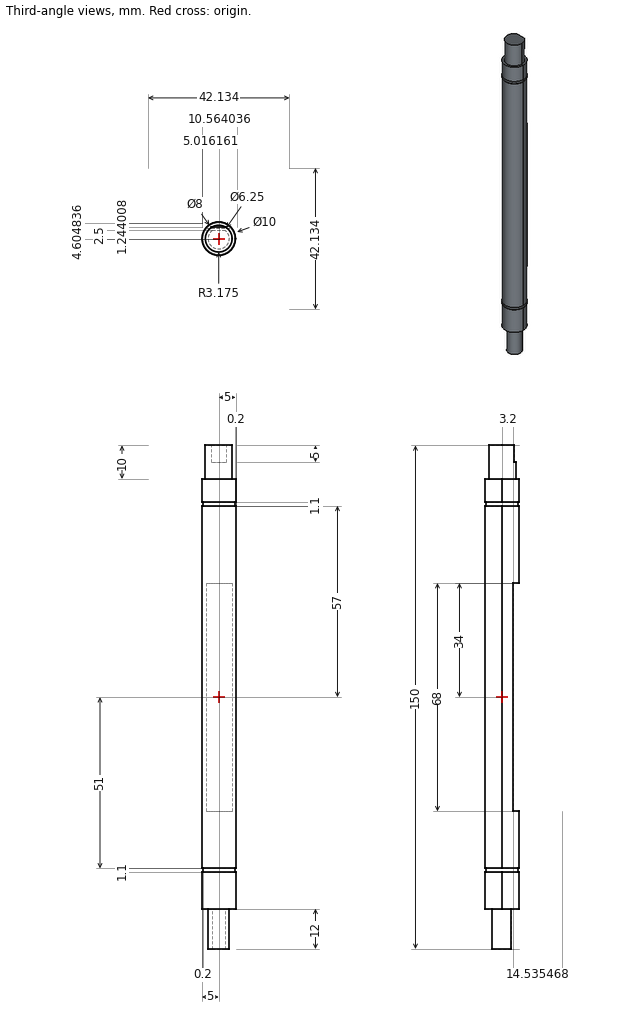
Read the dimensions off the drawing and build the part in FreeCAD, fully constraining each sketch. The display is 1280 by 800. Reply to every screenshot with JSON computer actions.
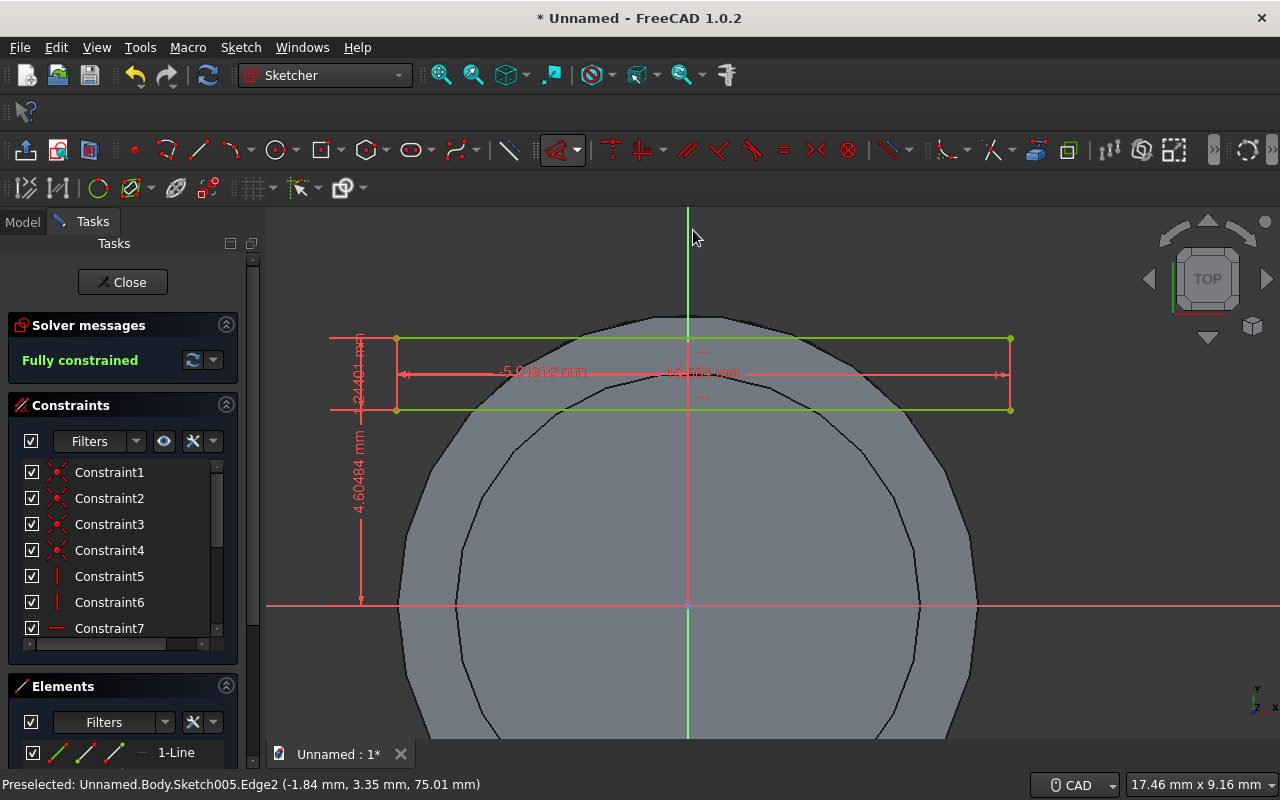
{"action": "left_click", "coordinate": [123, 282]}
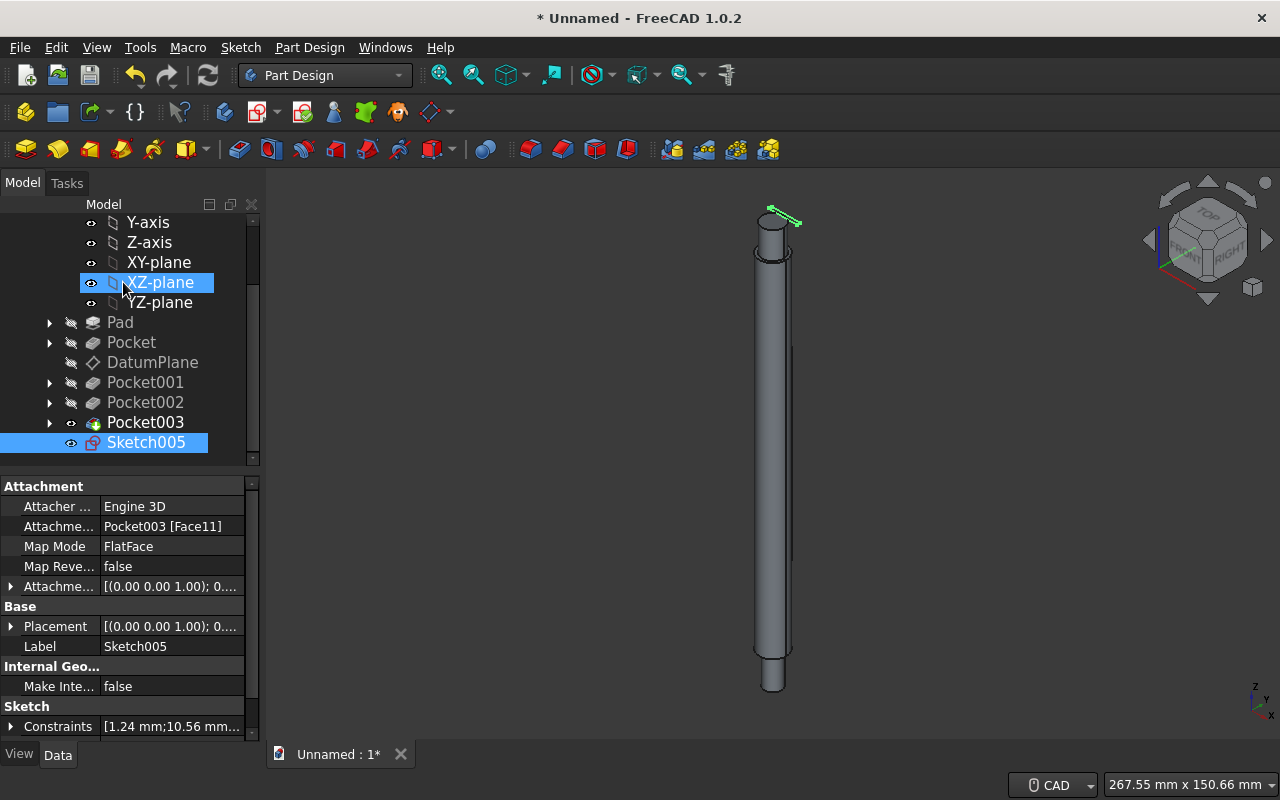
{"action": "left_click", "coordinate": [240, 150]}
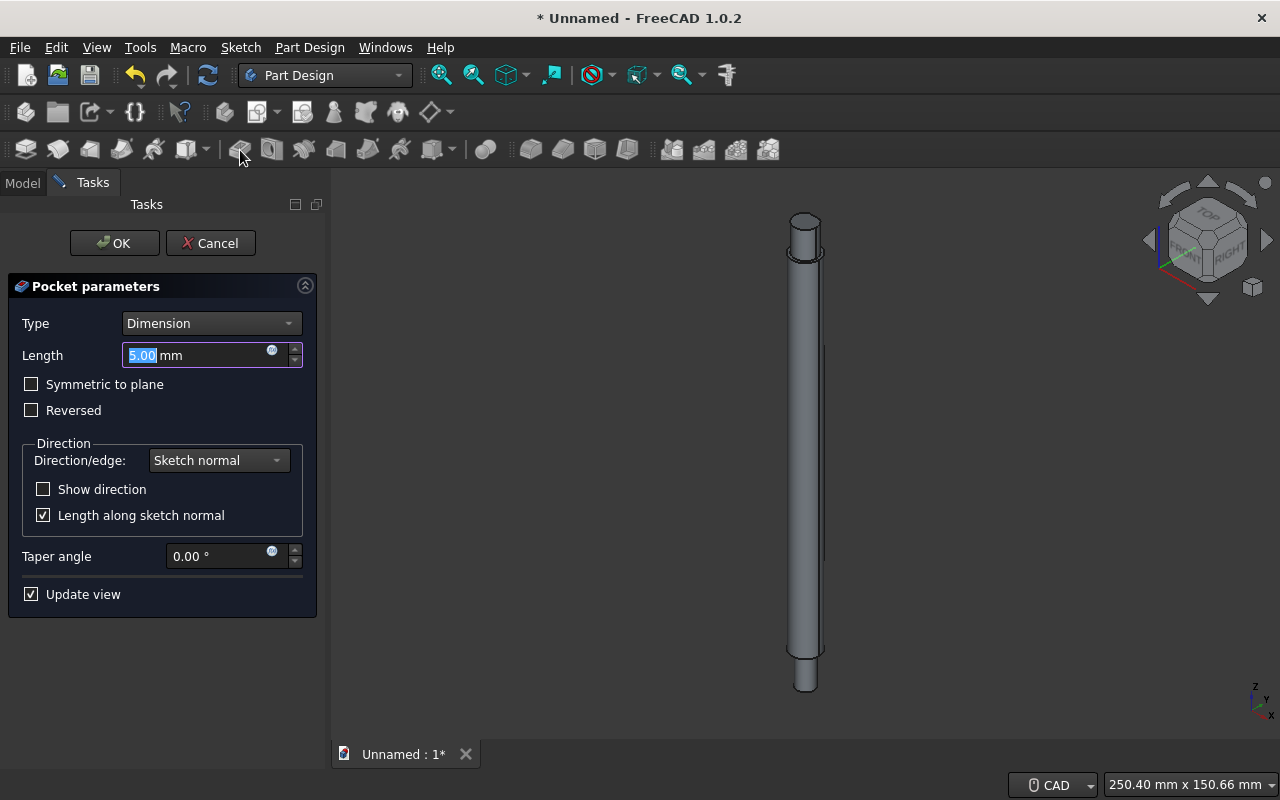
{"action": "type", "text": "5"}
{"action": "key", "text": "Tab"}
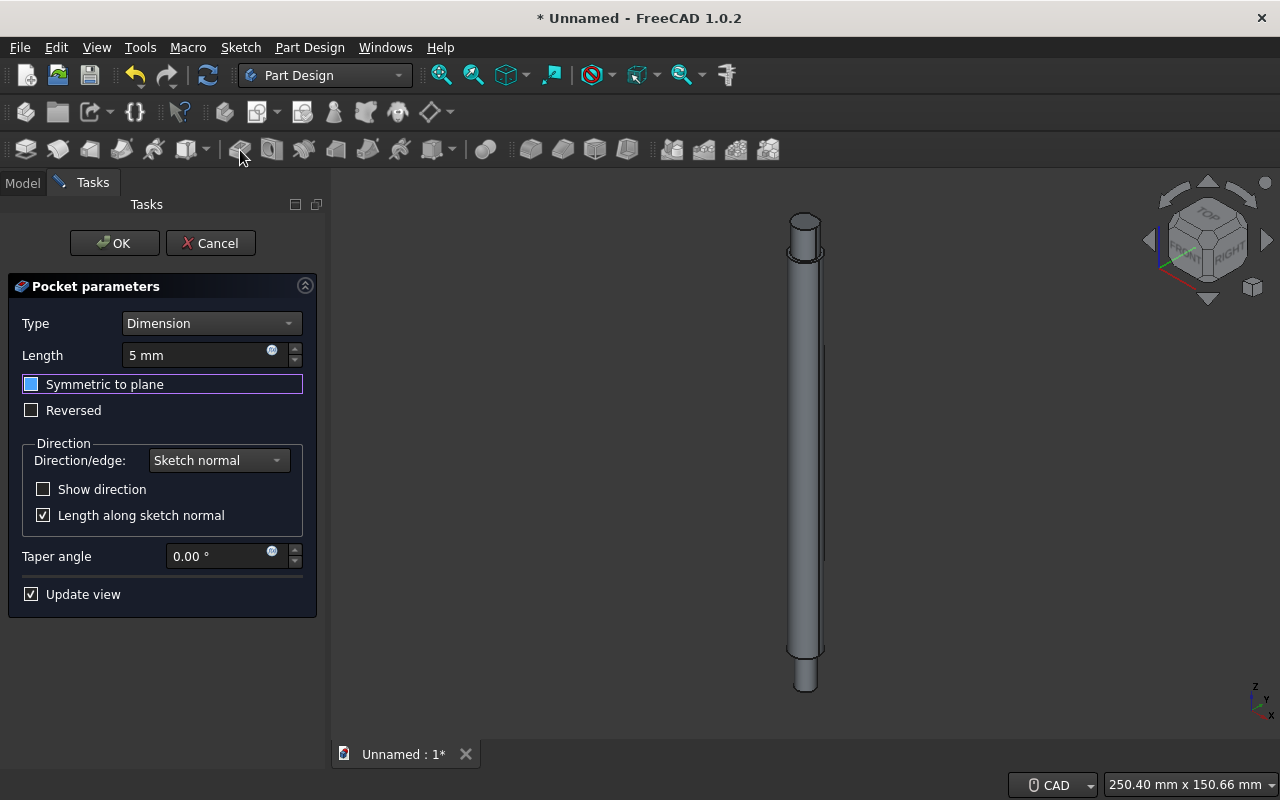
{"action": "left_click", "coordinate": [115, 243]}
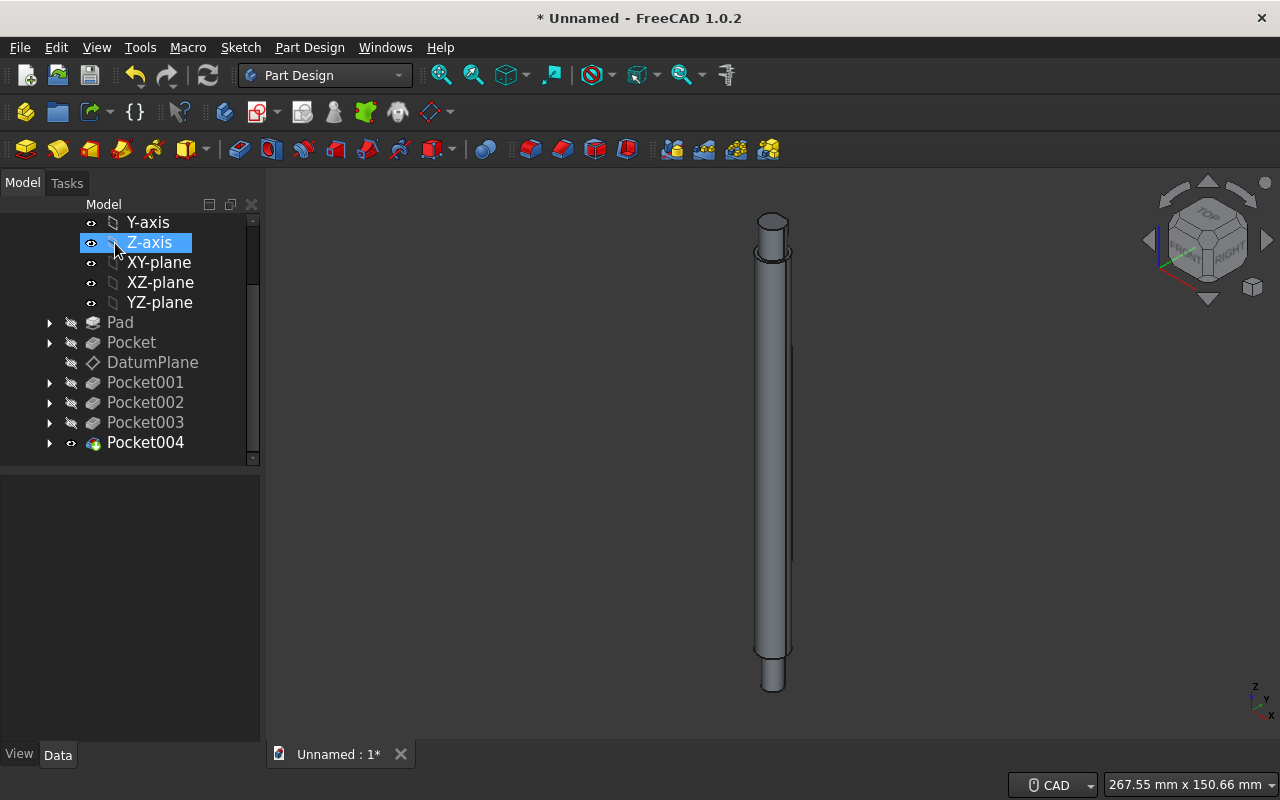
{"action": "left_click", "coordinate": [258, 112]}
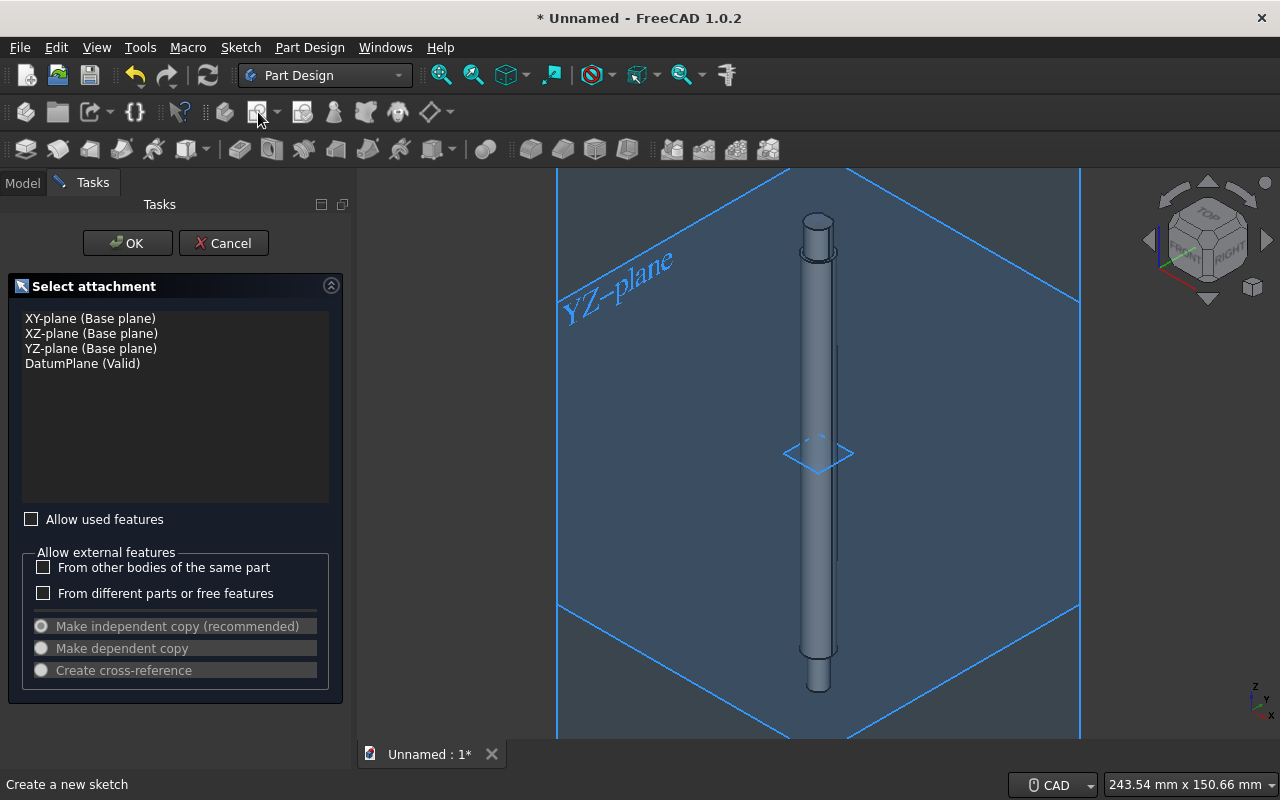
{"action": "left_click", "coordinate": [82, 334]}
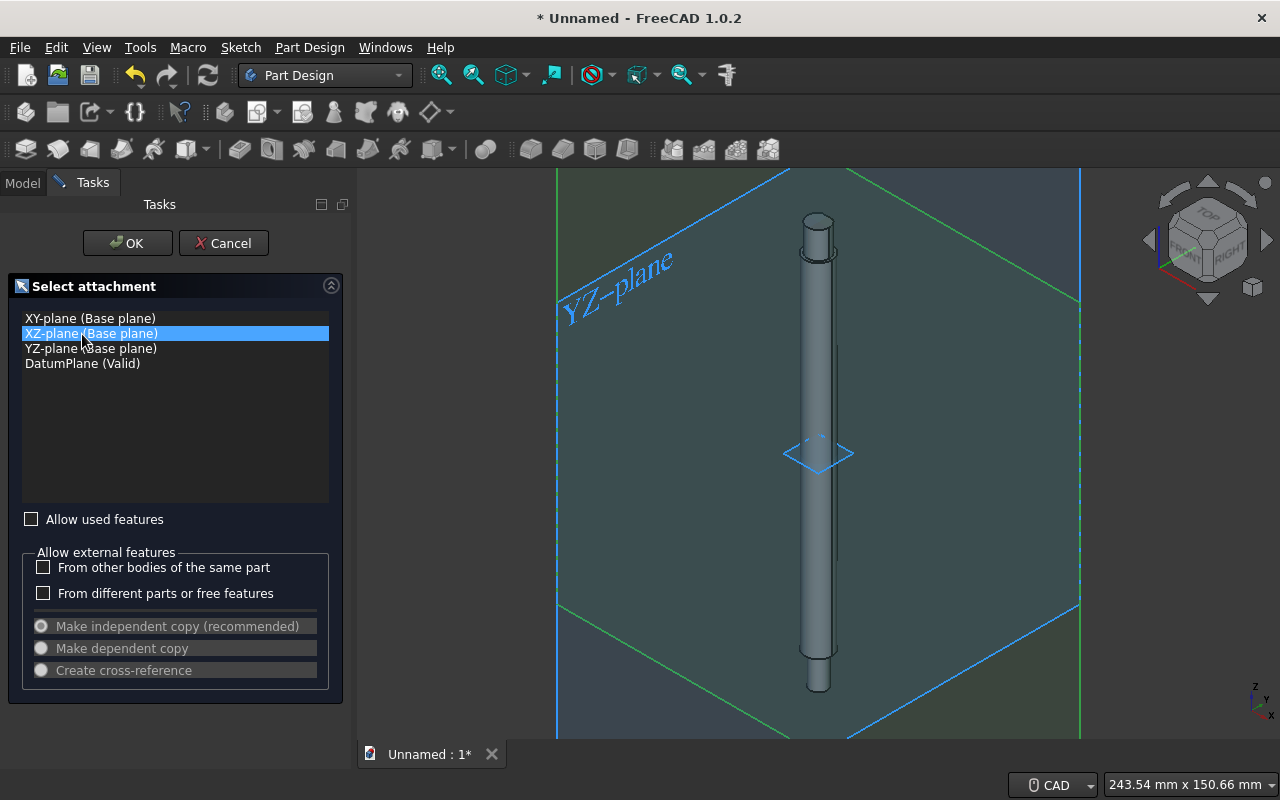
{"action": "left_click", "coordinate": [128, 243]}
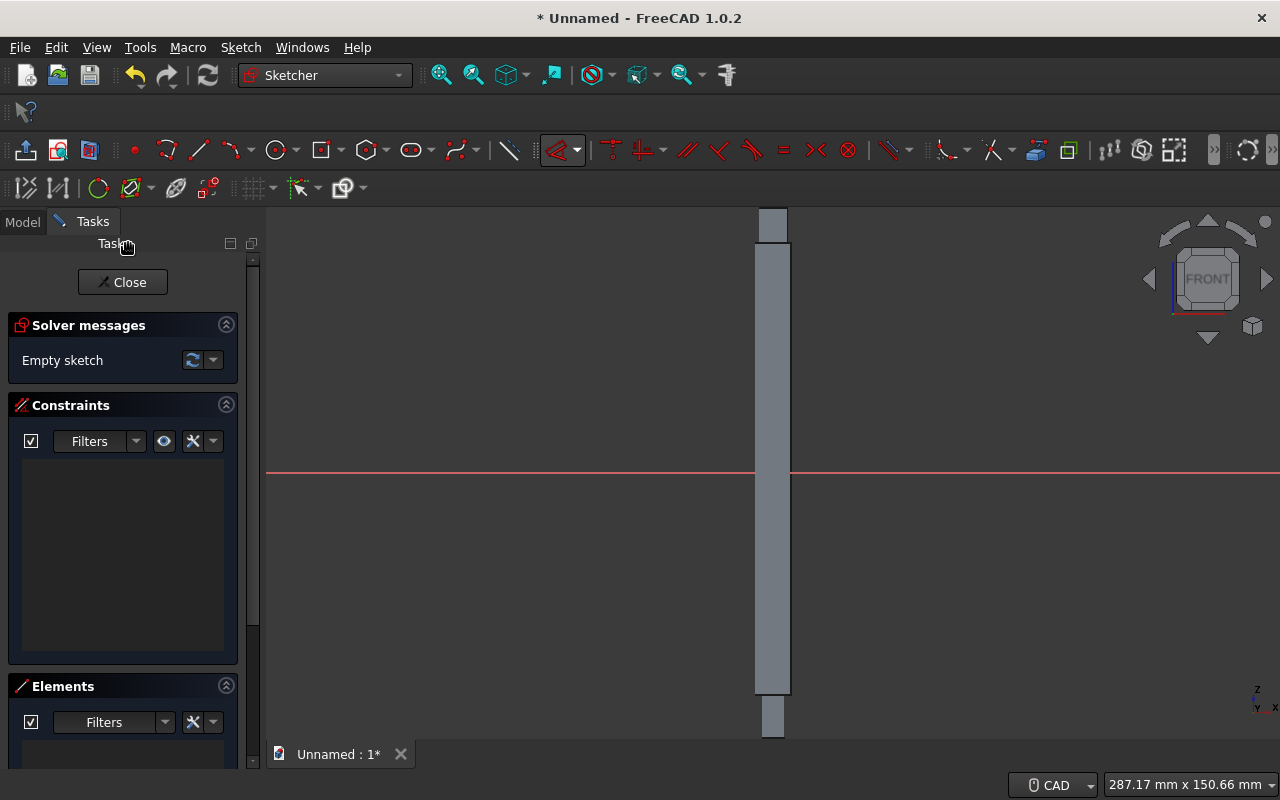
{"action": "left_click", "coordinate": [90, 150]}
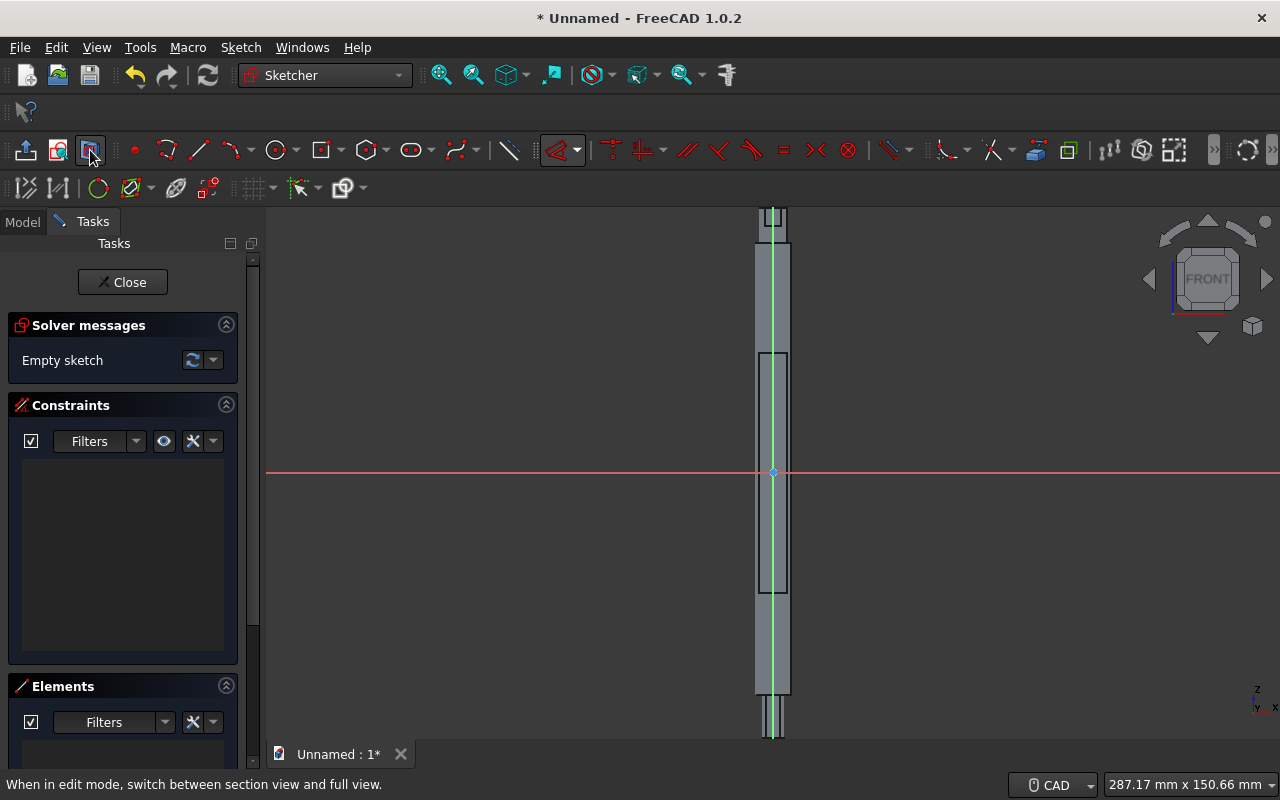
{"action": "scroll", "coordinate": [758, 665], "scroll_direction": "up", "scroll_amount": 15}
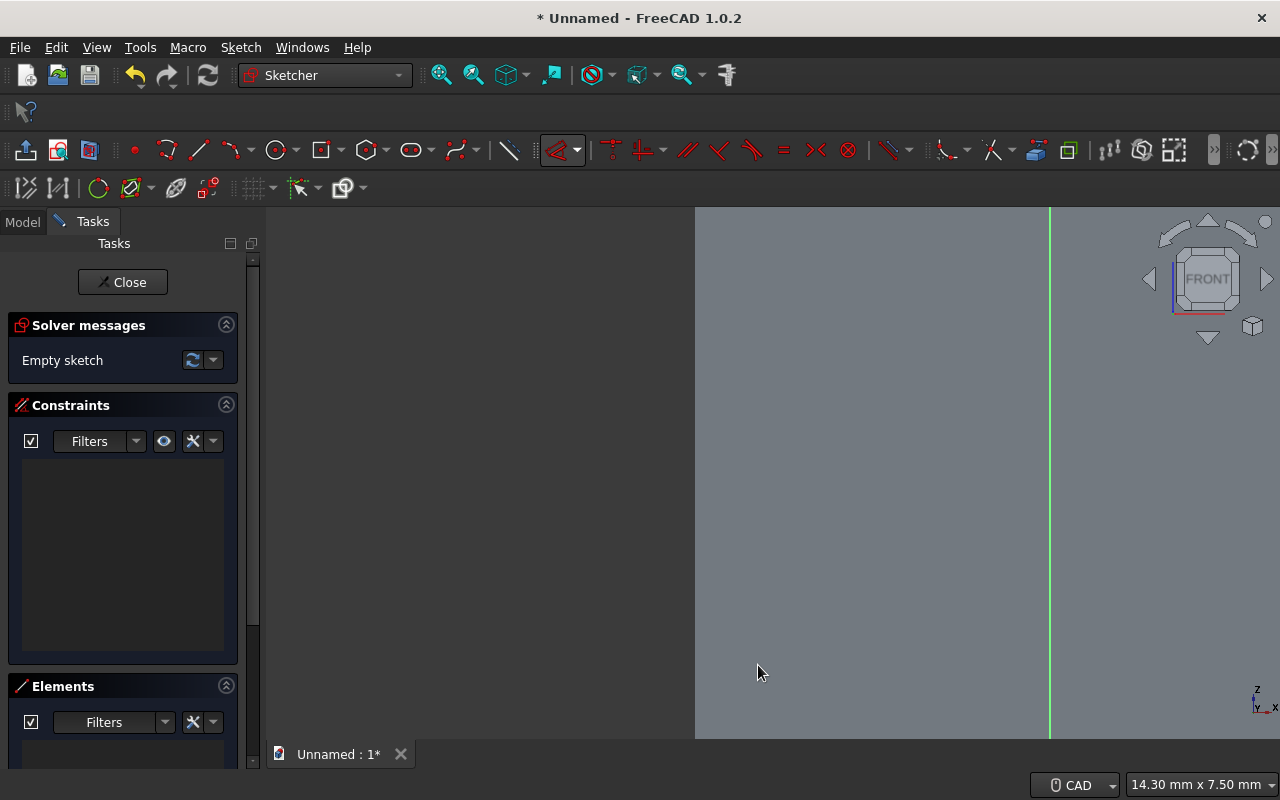
{"action": "scroll", "coordinate": [702, 440], "scroll_direction": "up", "scroll_amount": 7}